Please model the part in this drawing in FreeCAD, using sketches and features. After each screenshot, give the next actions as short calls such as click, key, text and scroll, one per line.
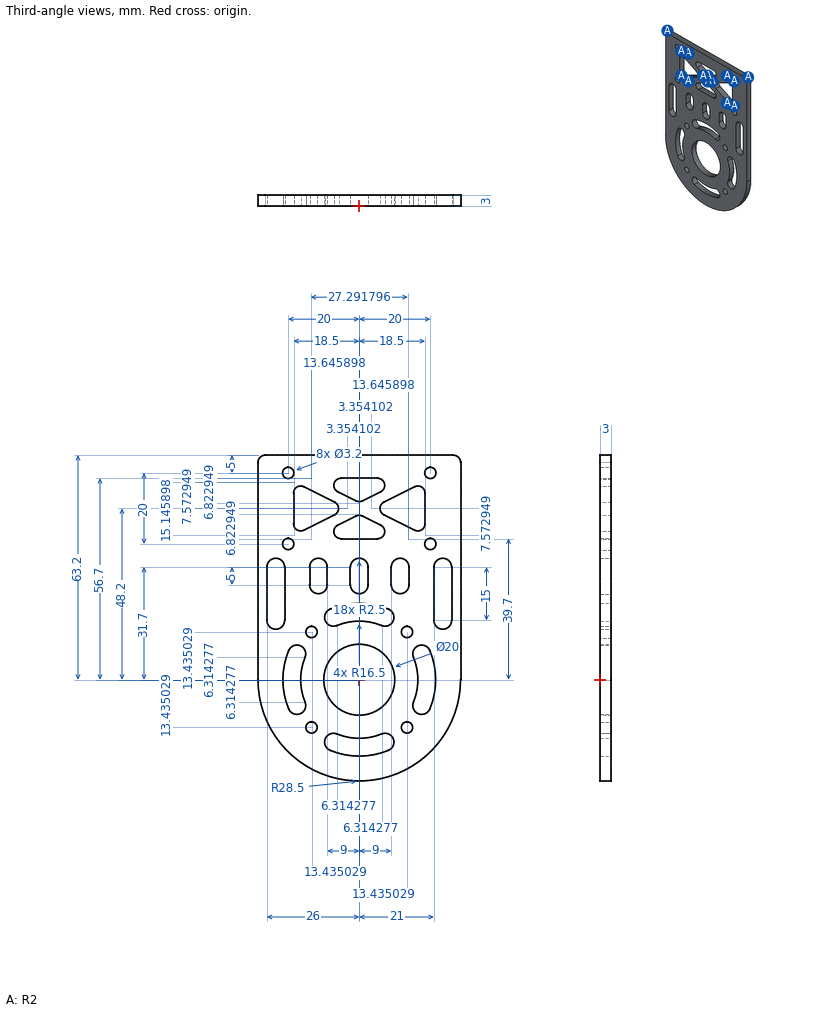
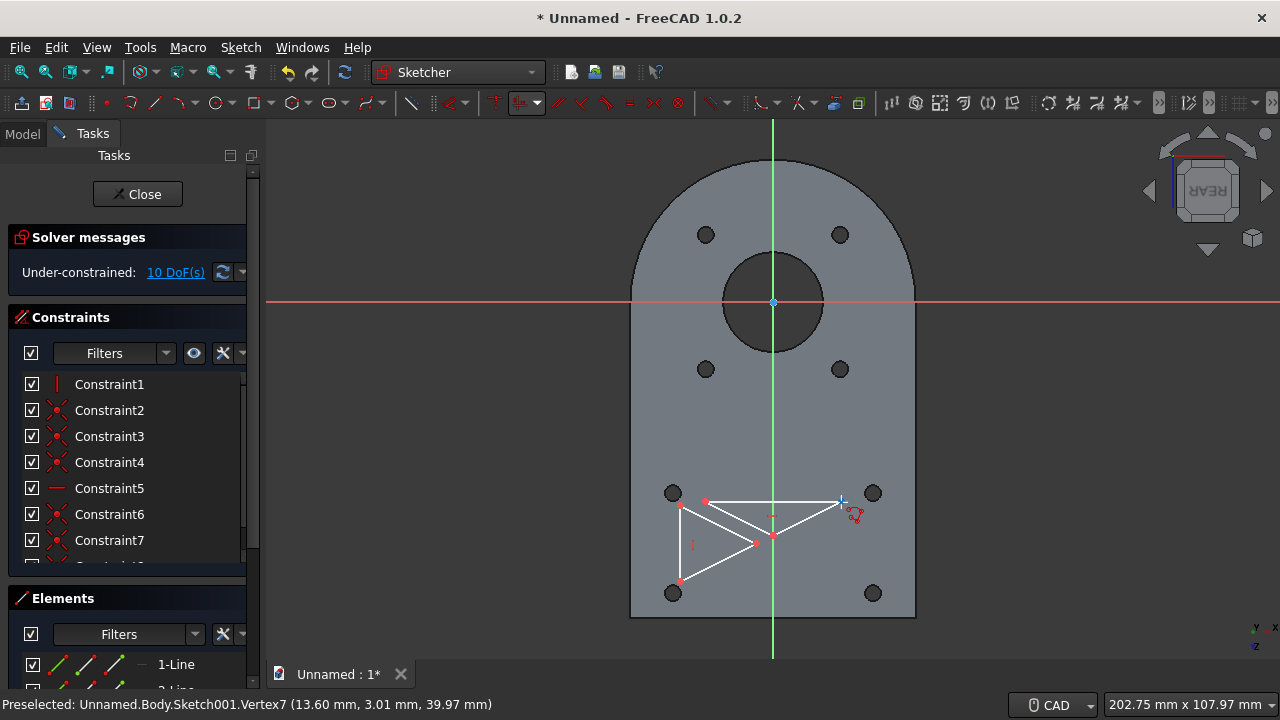
click(866, 505)
click(790, 543)
click(866, 581)
click(866, 506)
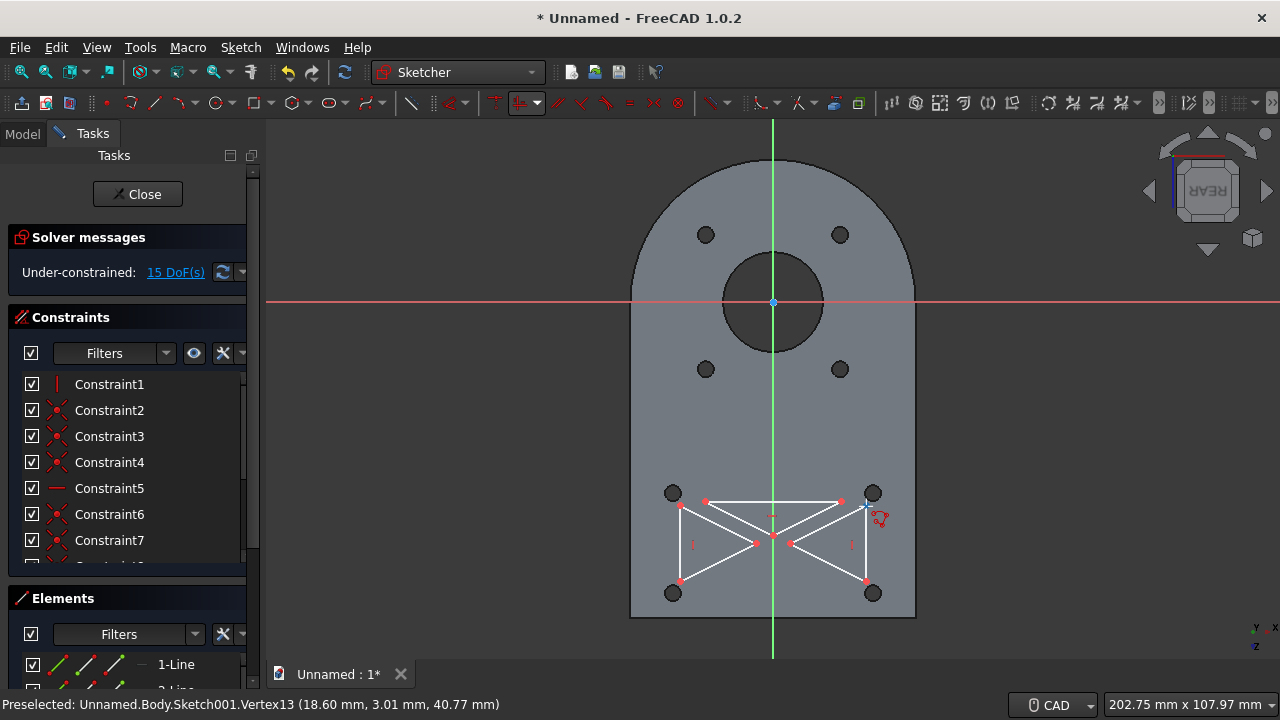
click(773, 552)
click(705, 586)
click(841, 586)
click(773, 553)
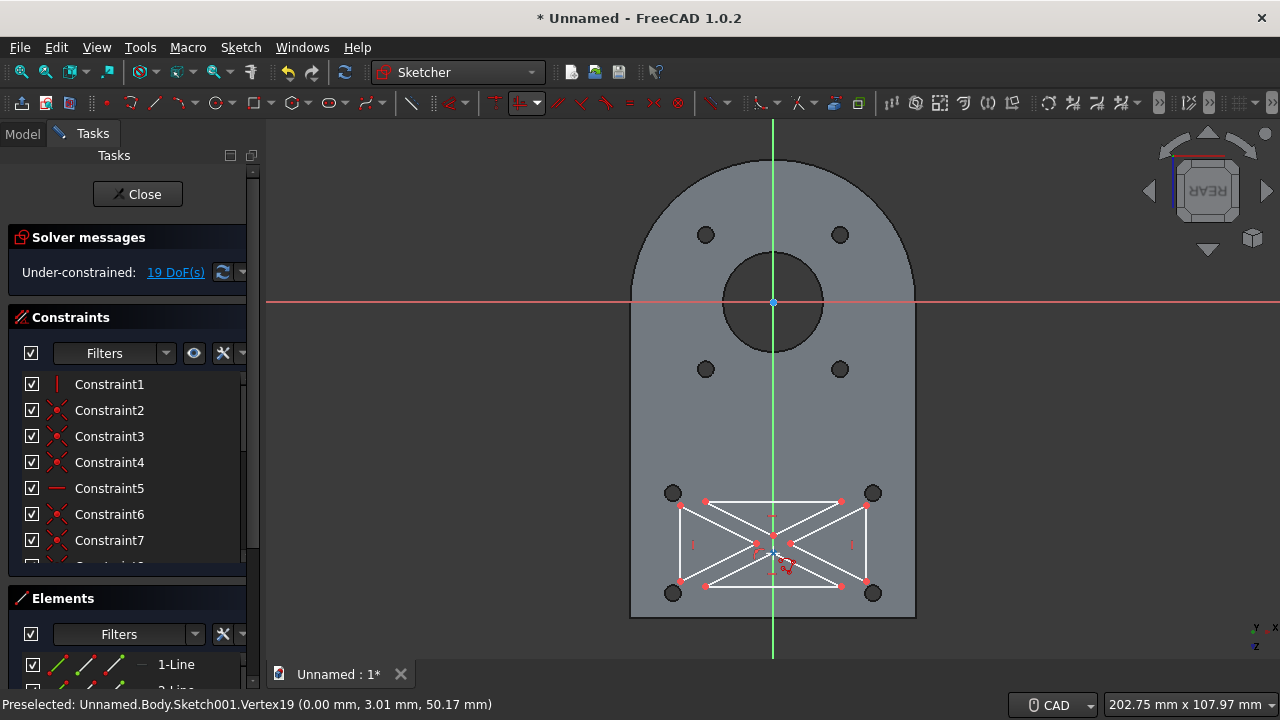
key(g)
key(s)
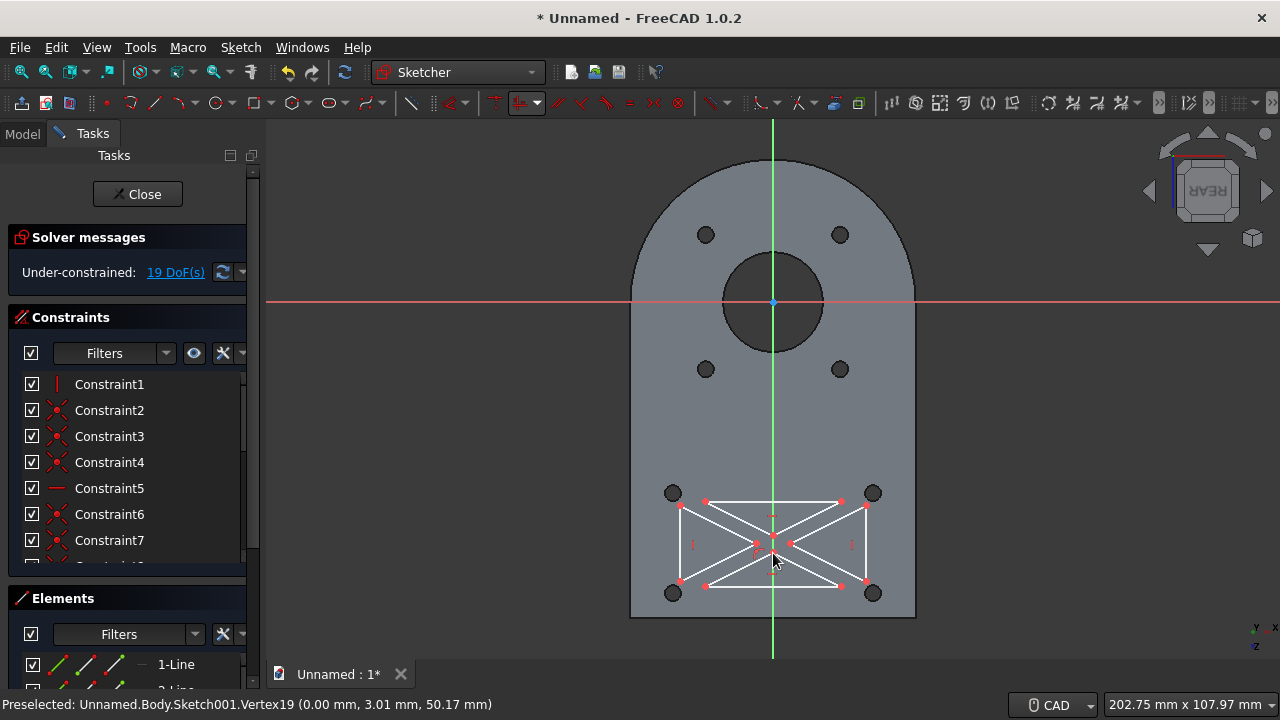
scroll(773, 461, up, 3)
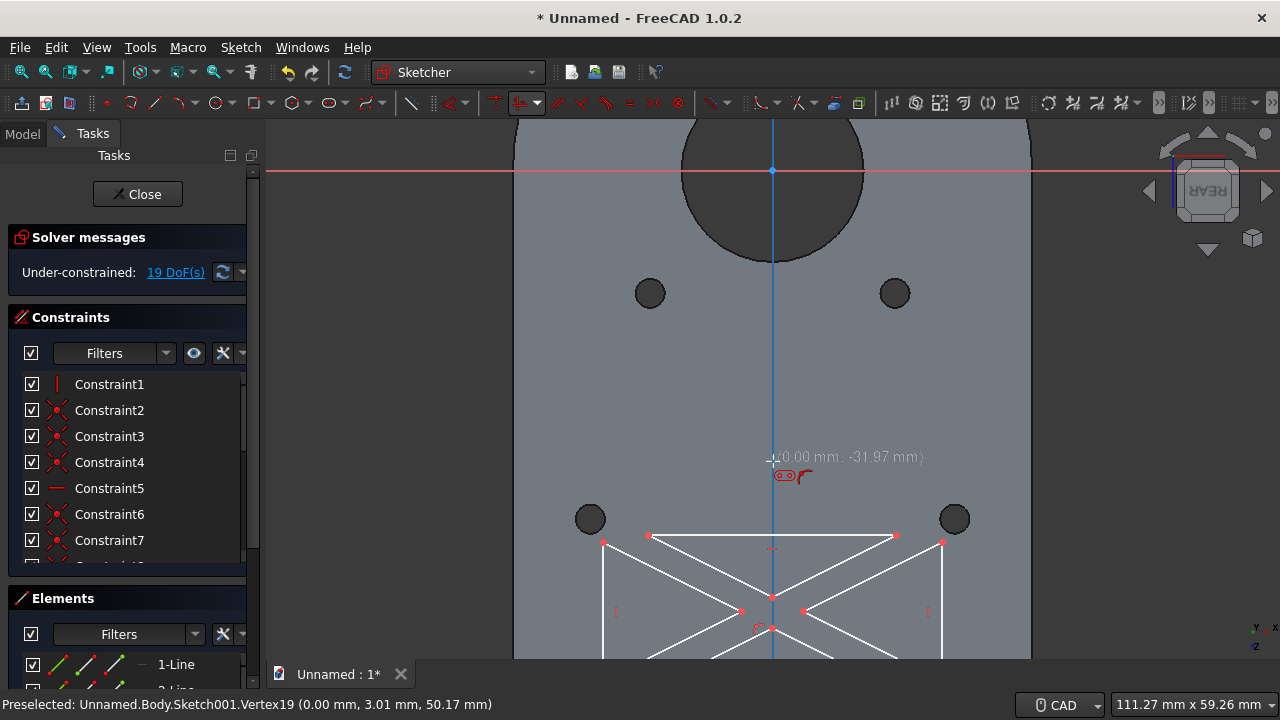
click(773, 460)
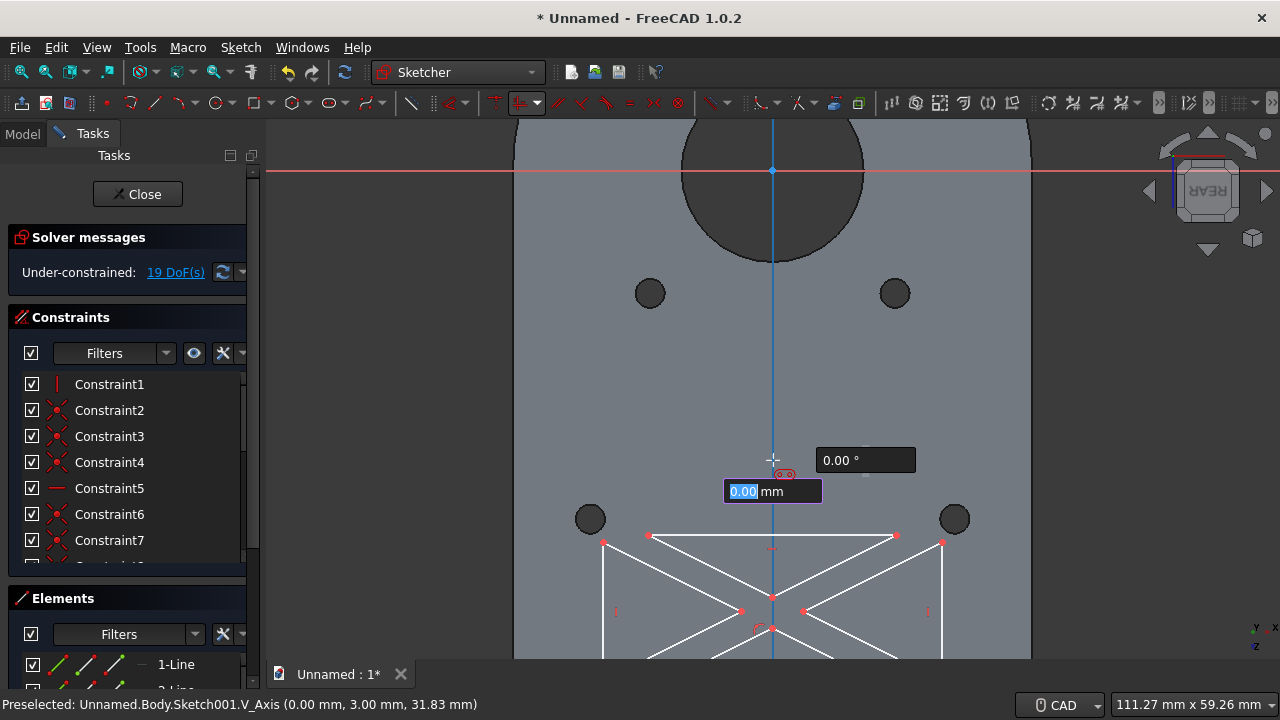
click(782, 414)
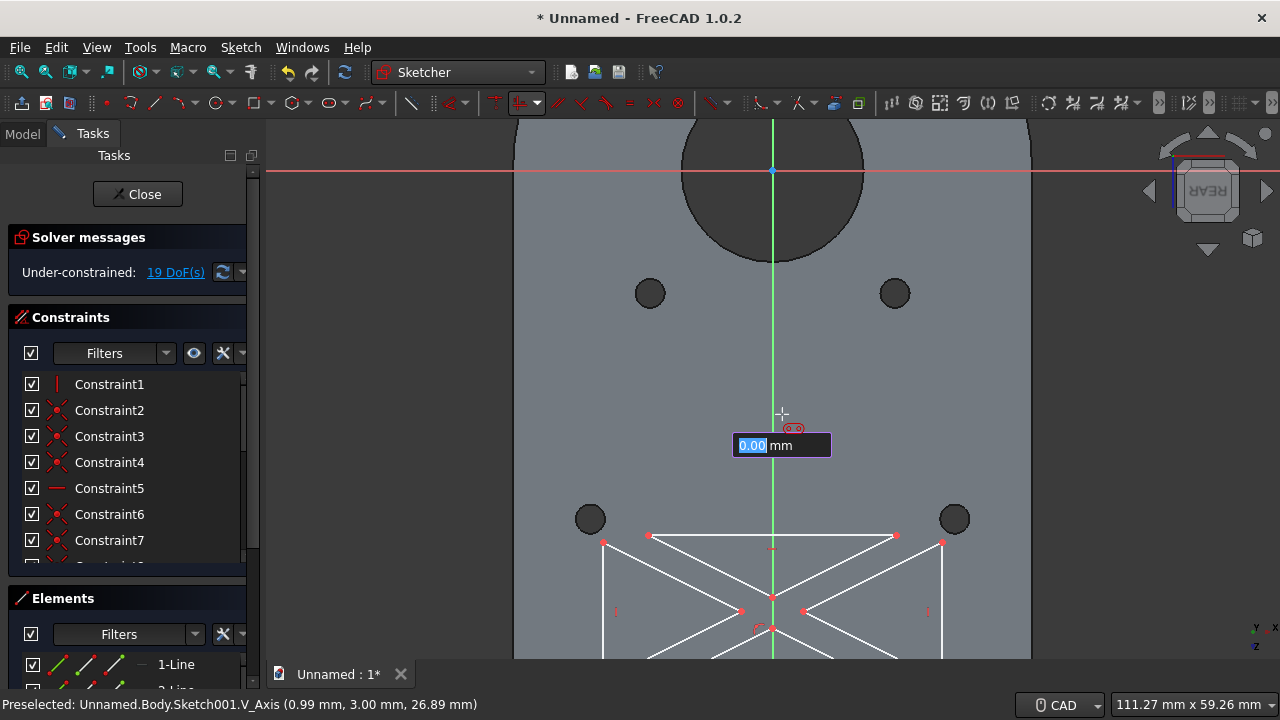
click(750, 437)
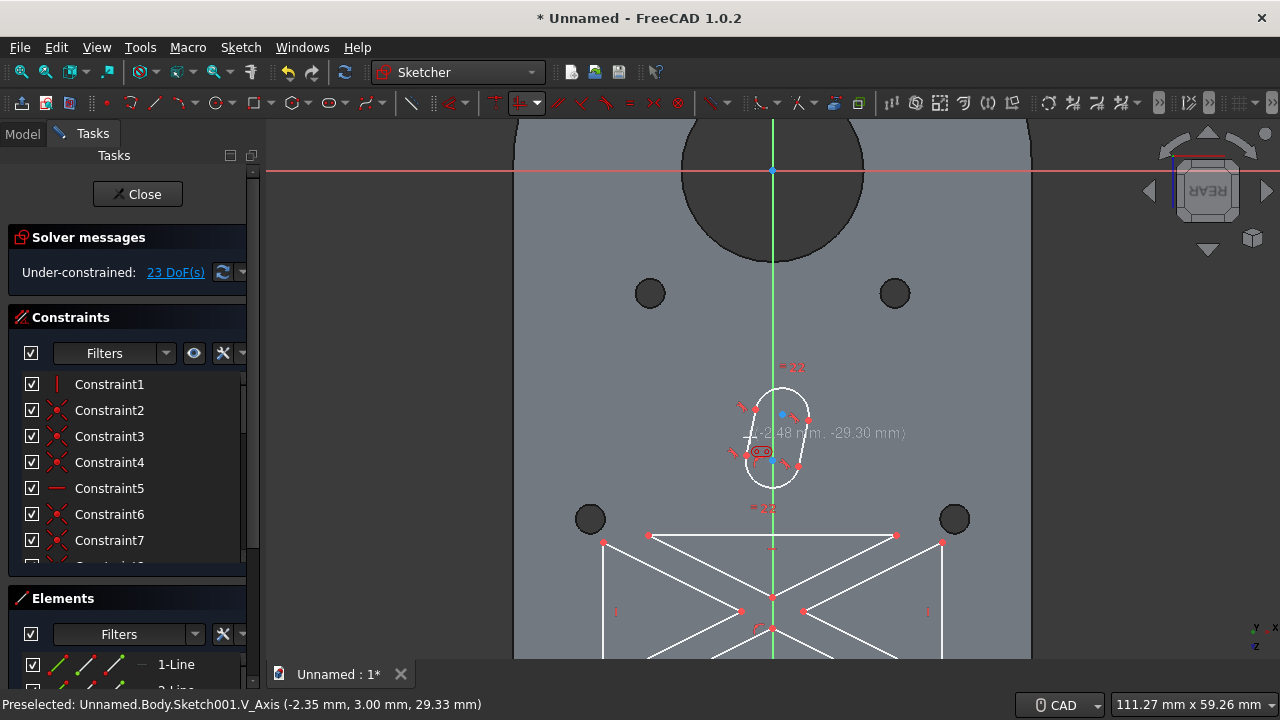
click(877, 460)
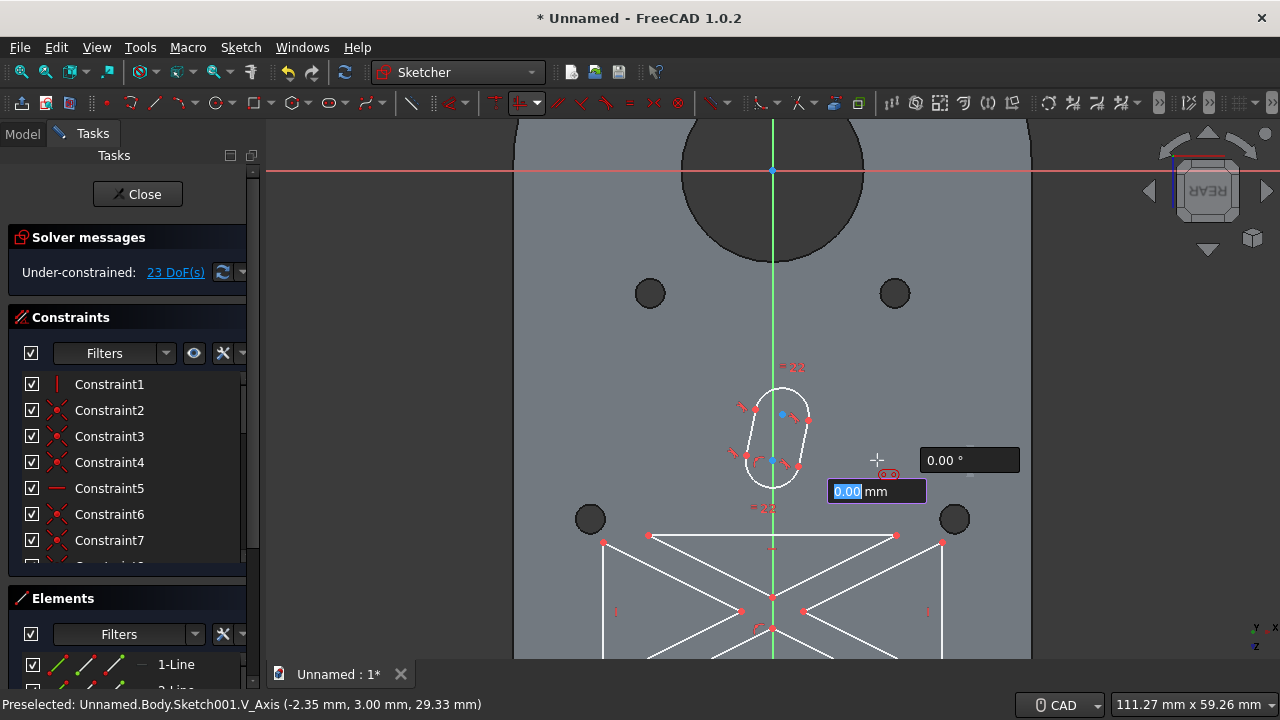
click(877, 414)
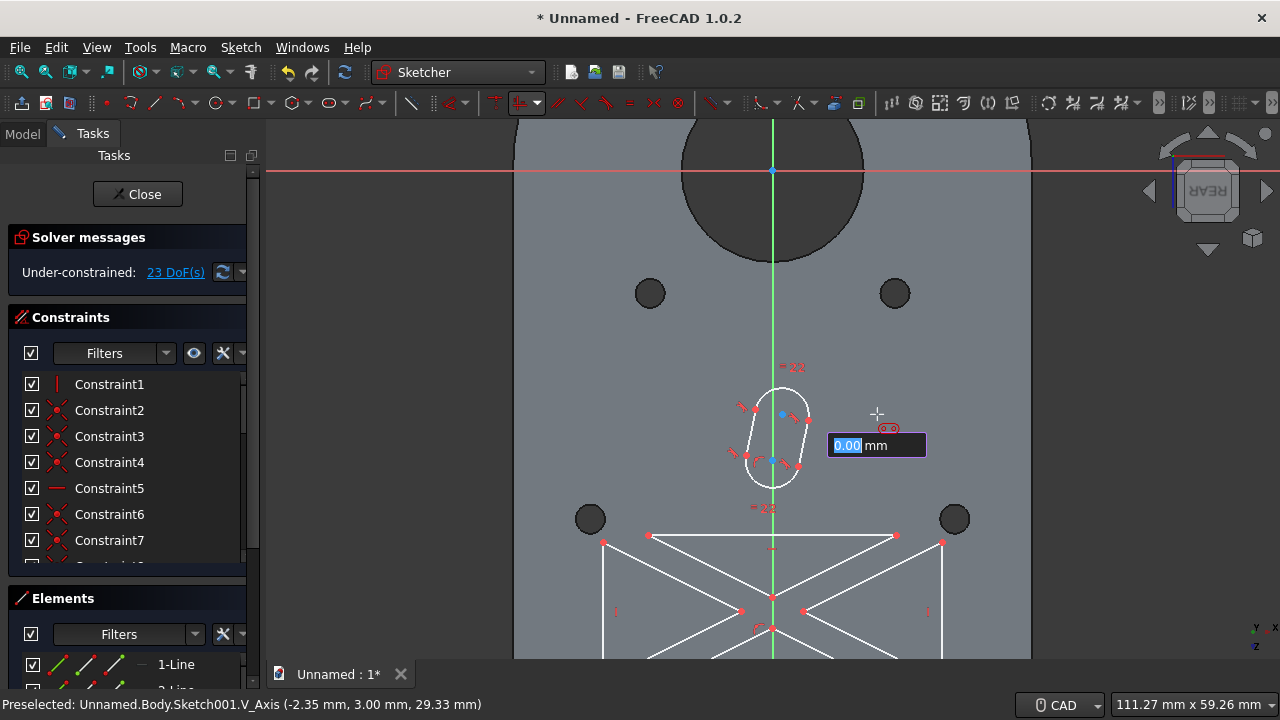
click(900, 437)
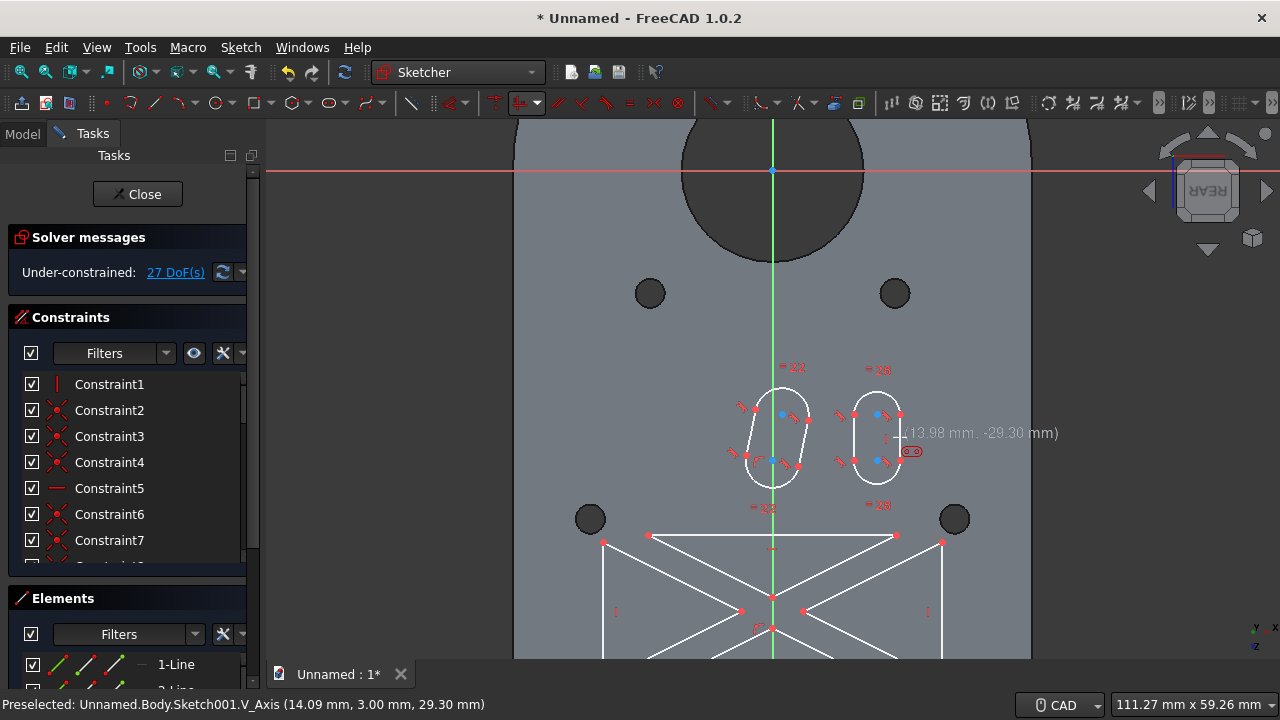
click(987, 460)